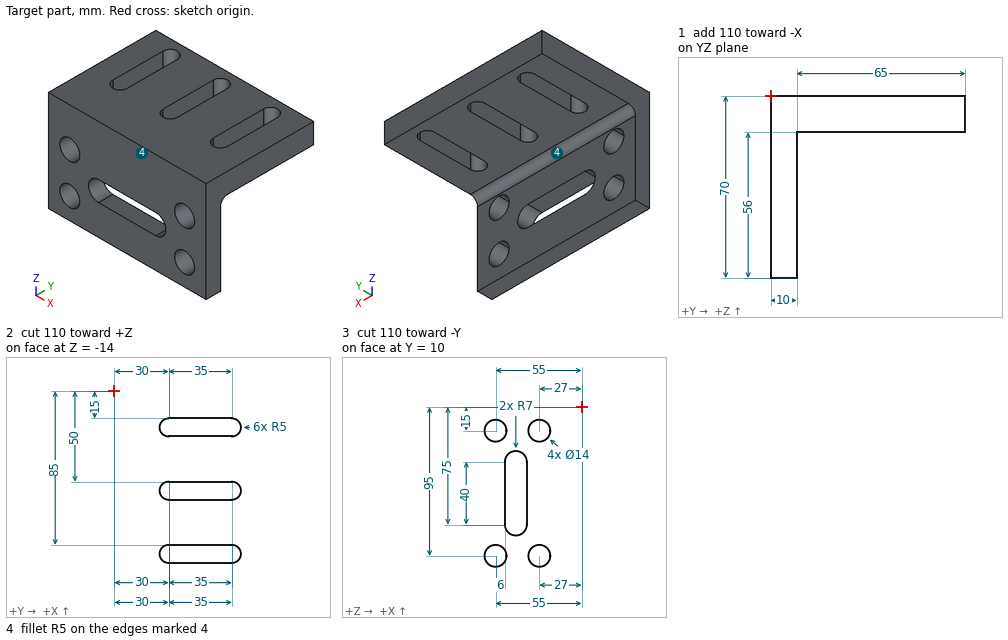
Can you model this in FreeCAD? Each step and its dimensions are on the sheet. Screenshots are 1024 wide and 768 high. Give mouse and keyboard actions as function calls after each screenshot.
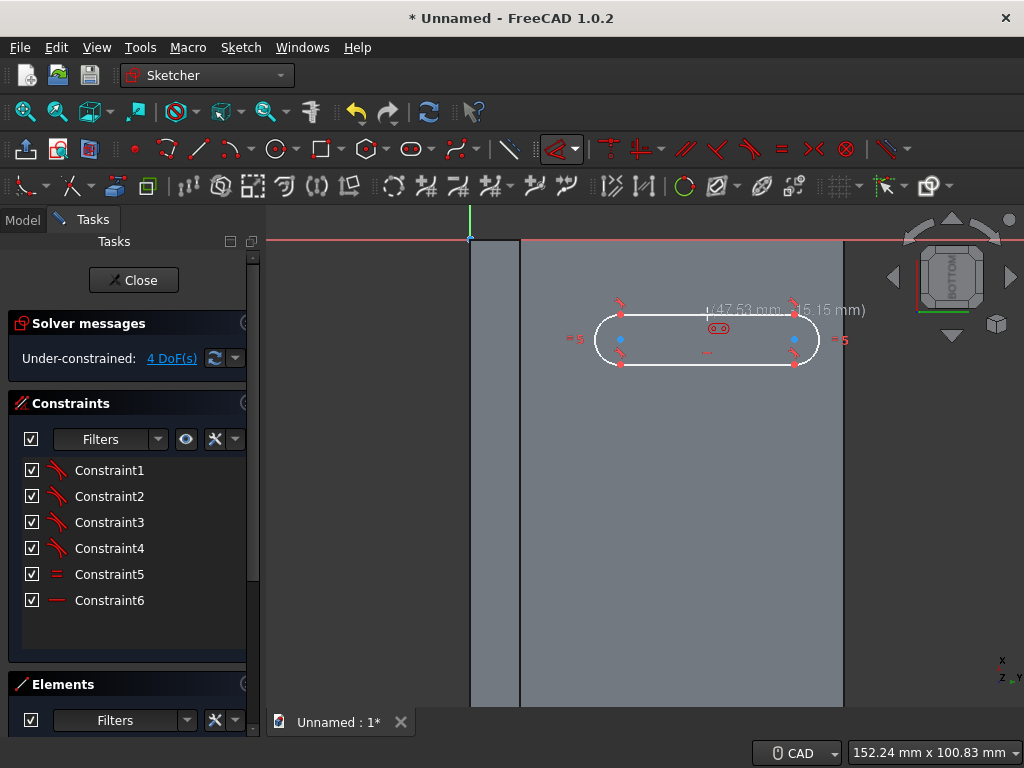
click(620, 513)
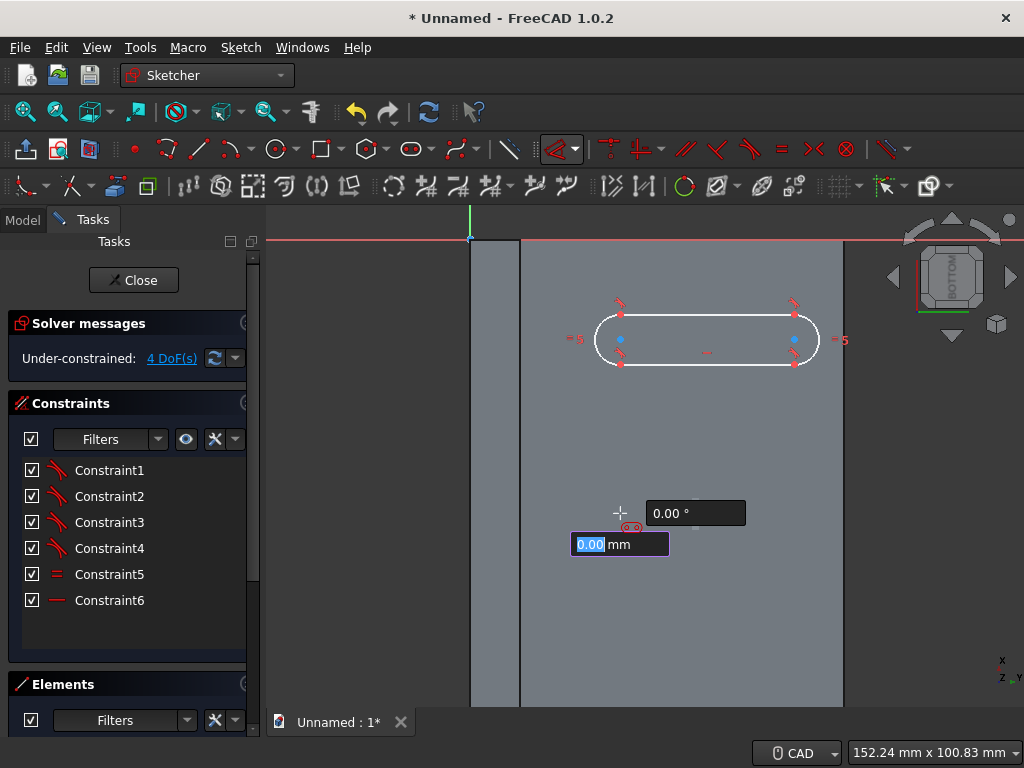
click(794, 513)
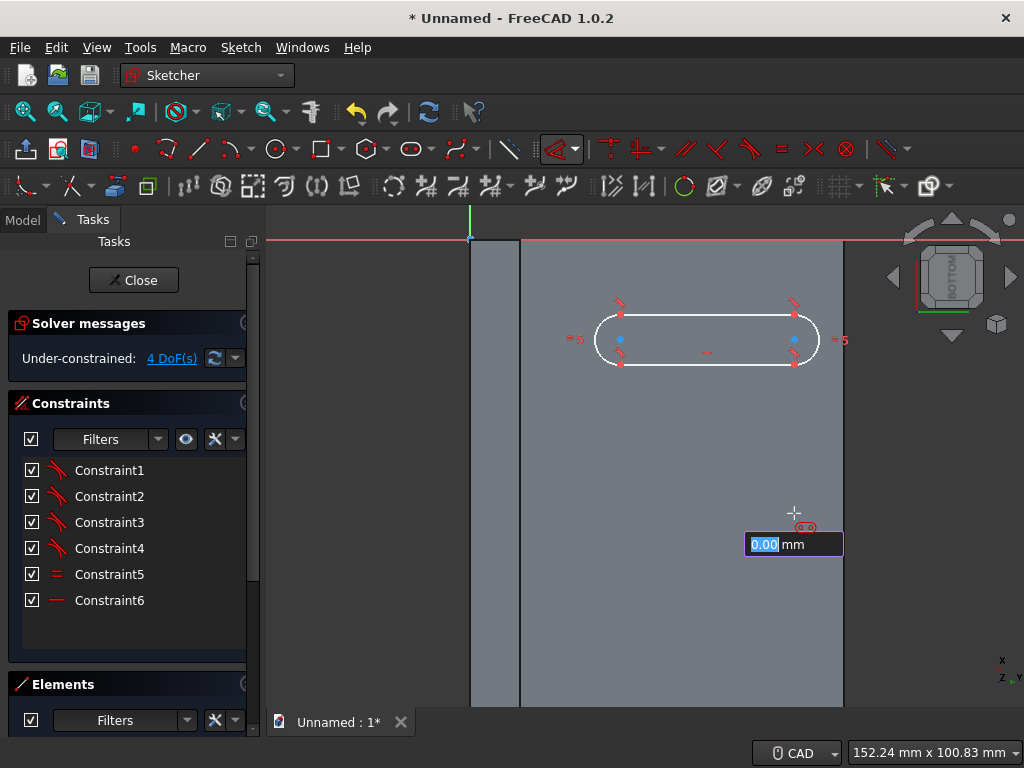
click(707, 489)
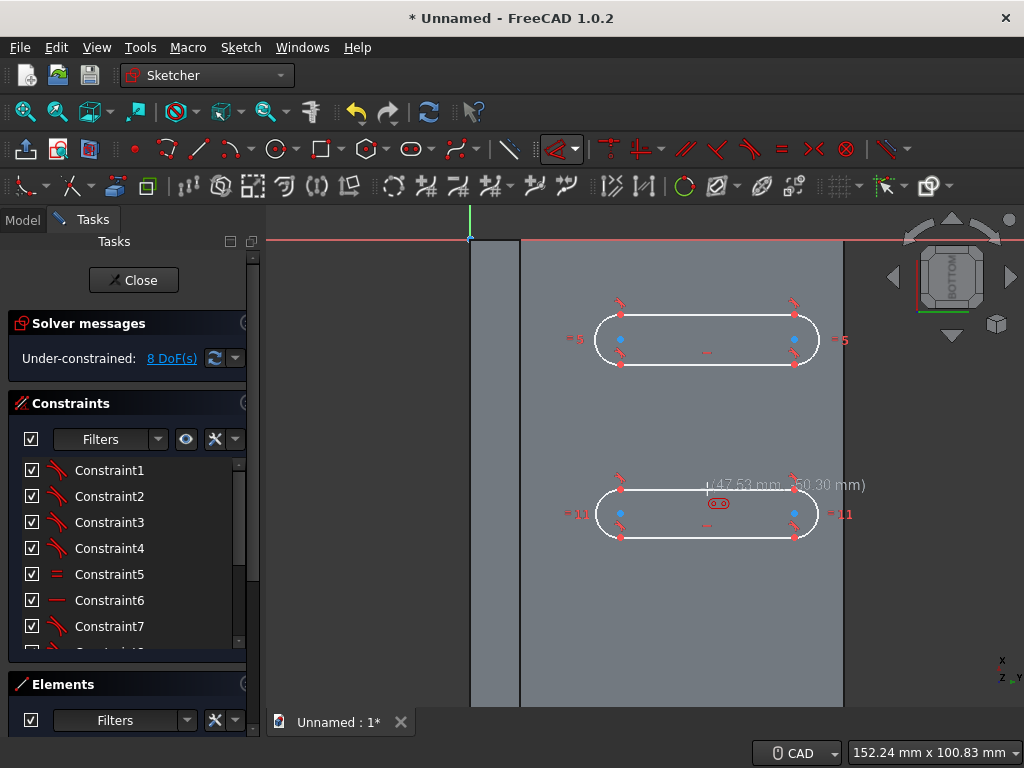
scroll(438, 415, down, 2)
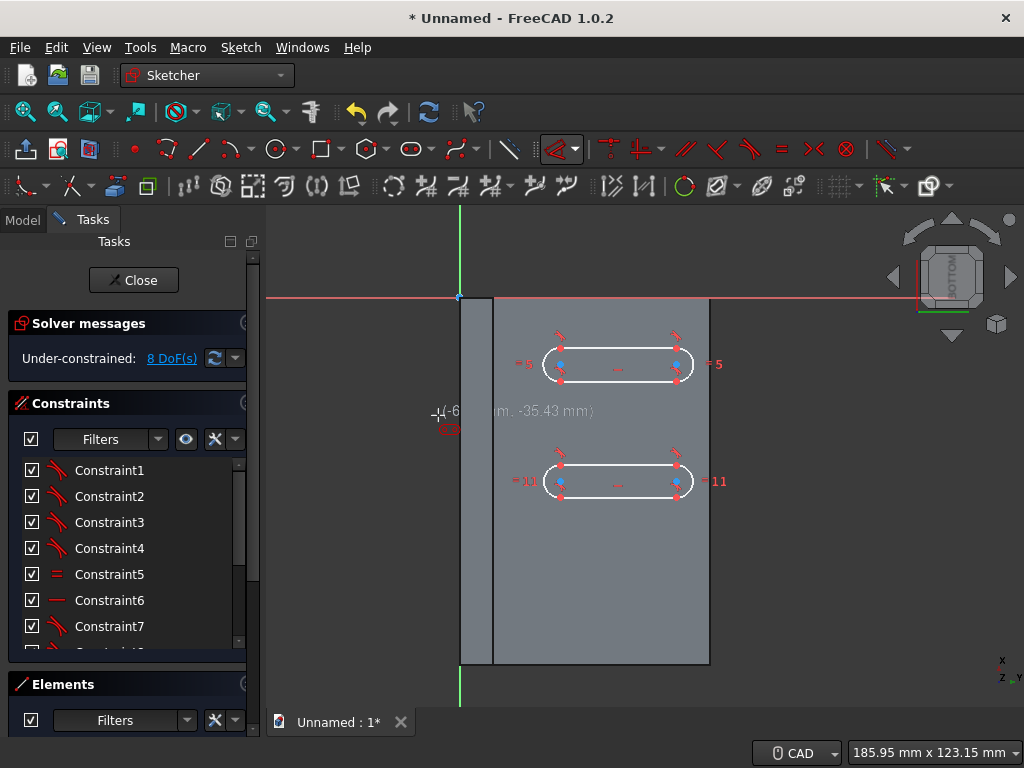
scroll(560, 598, up, 2)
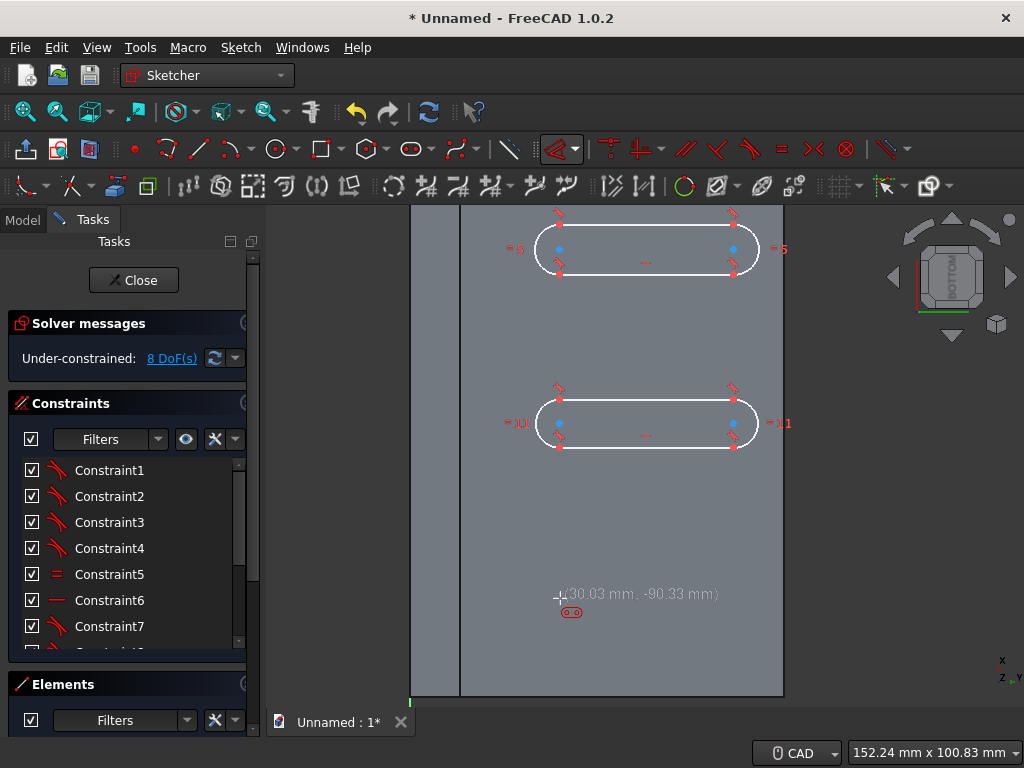
click(560, 597)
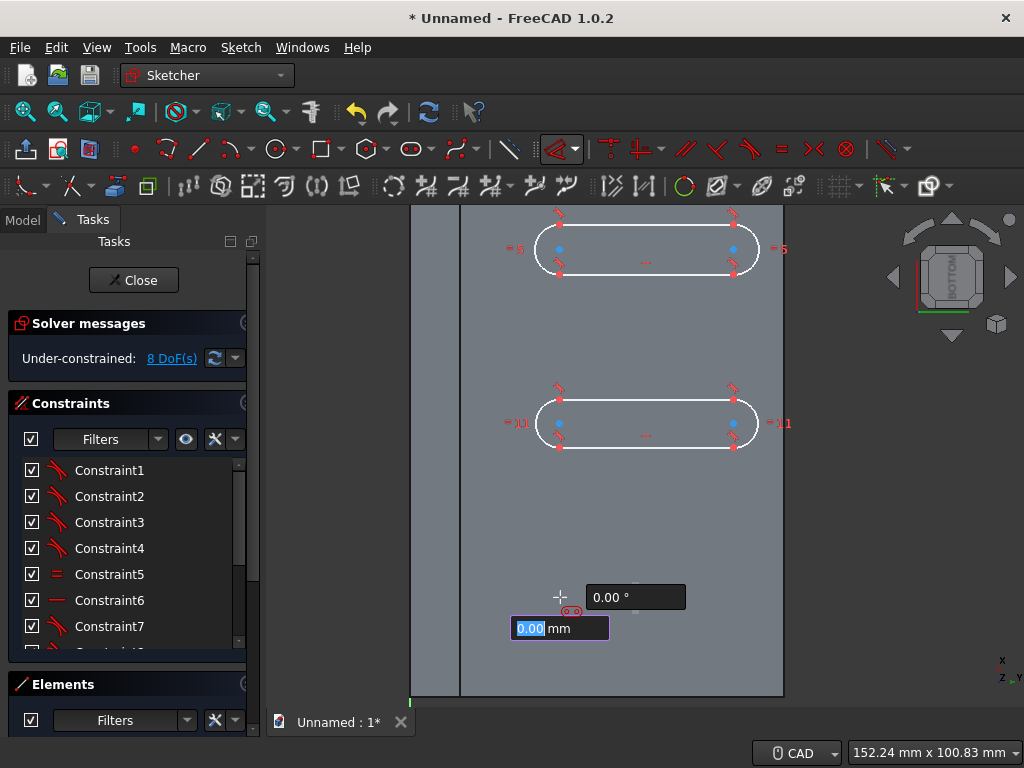
click(734, 597)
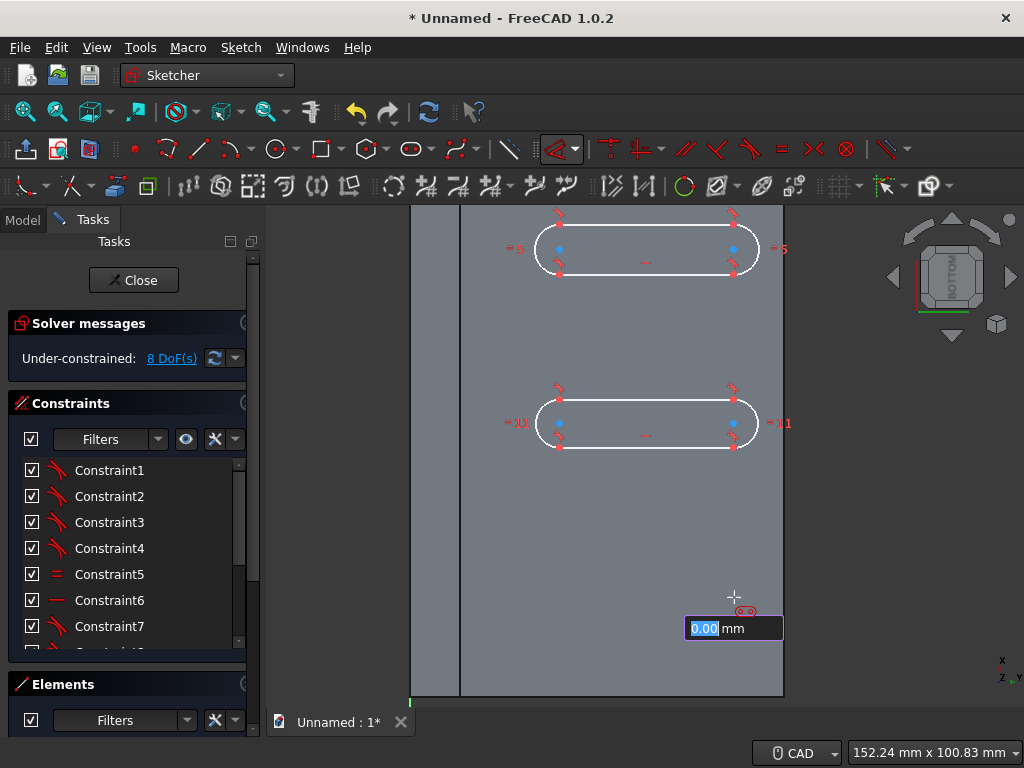
click(647, 573)
key(Escape)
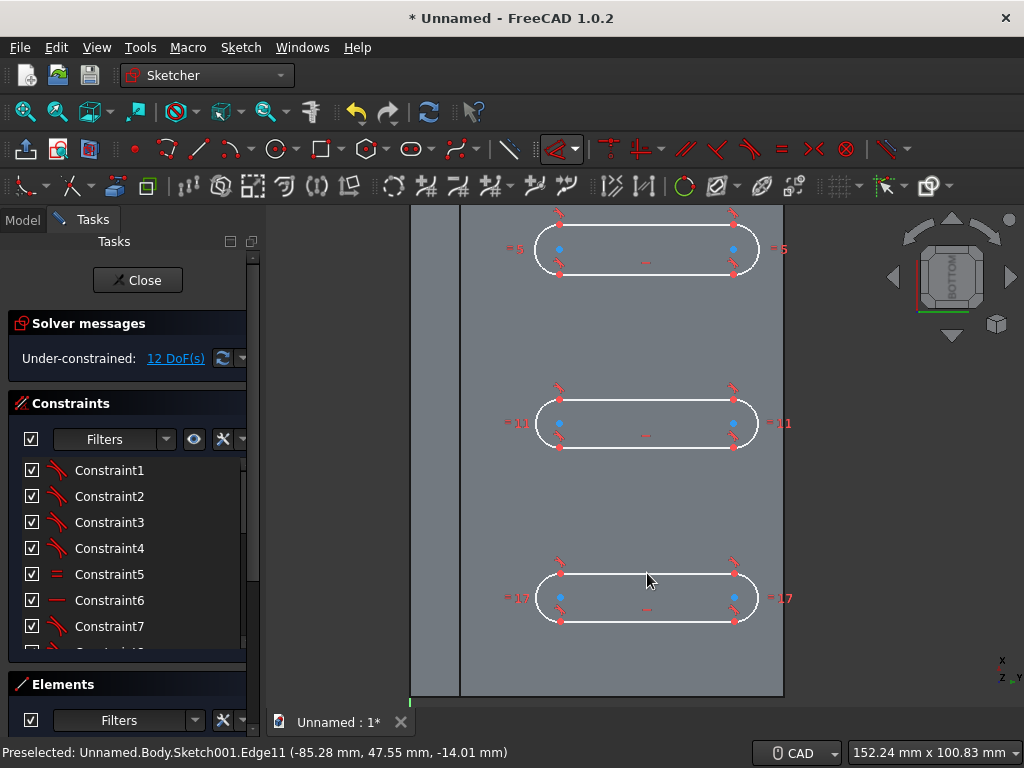
click(540, 235)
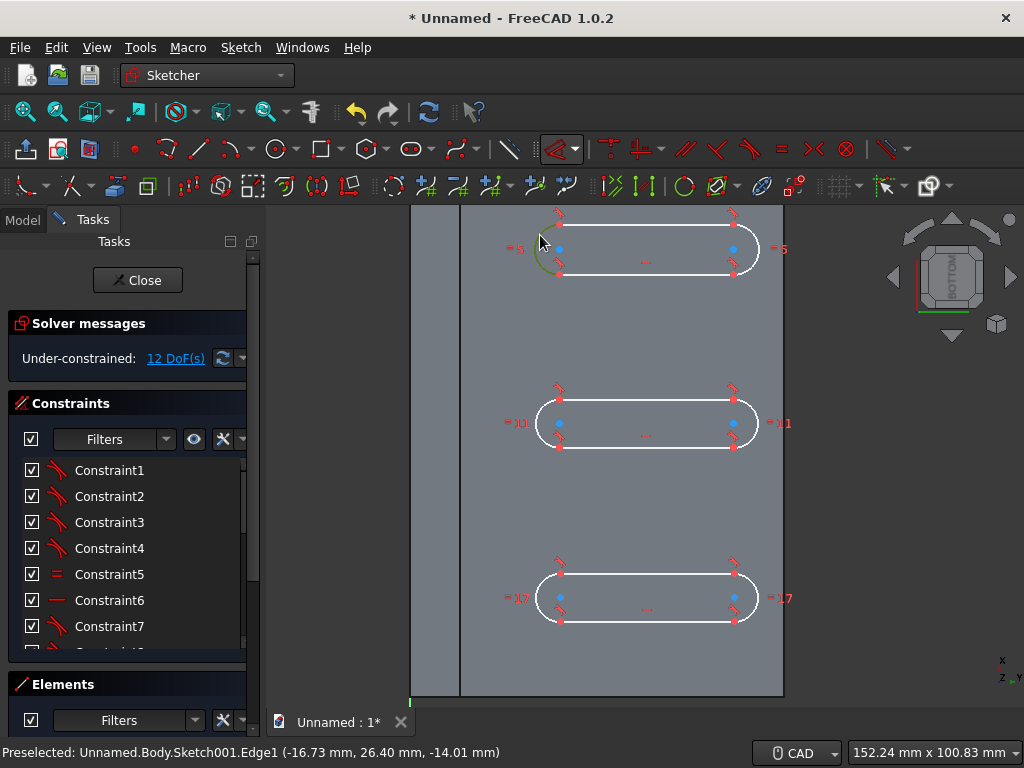
click(541, 410)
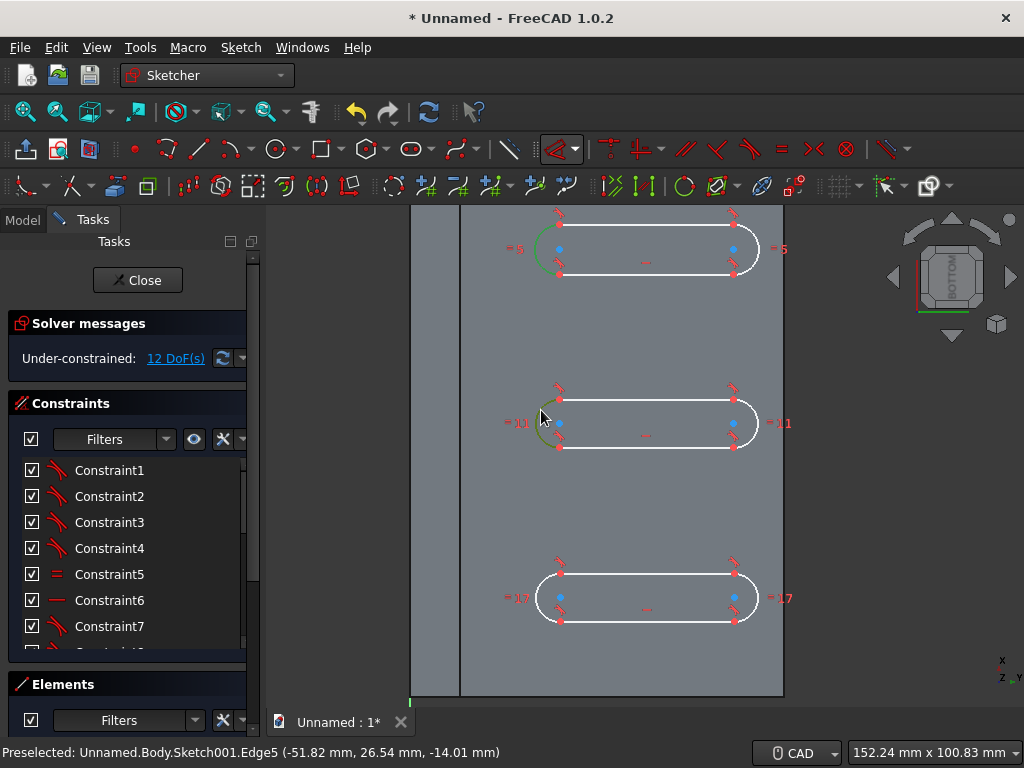
click(541, 584)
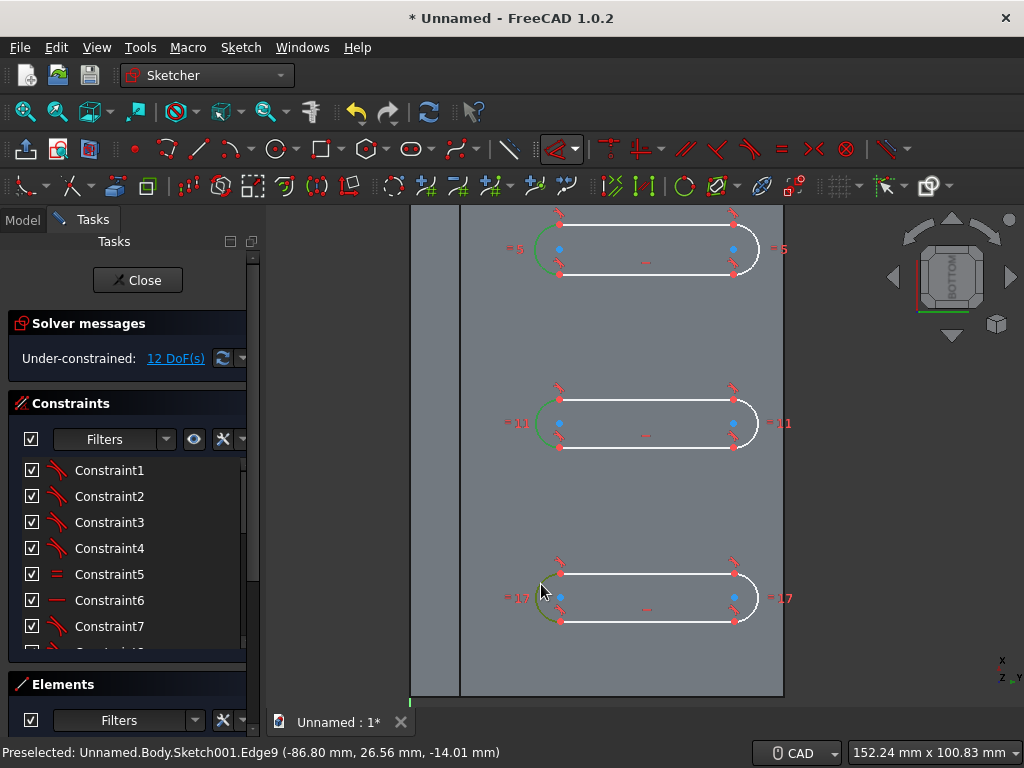
click(782, 150)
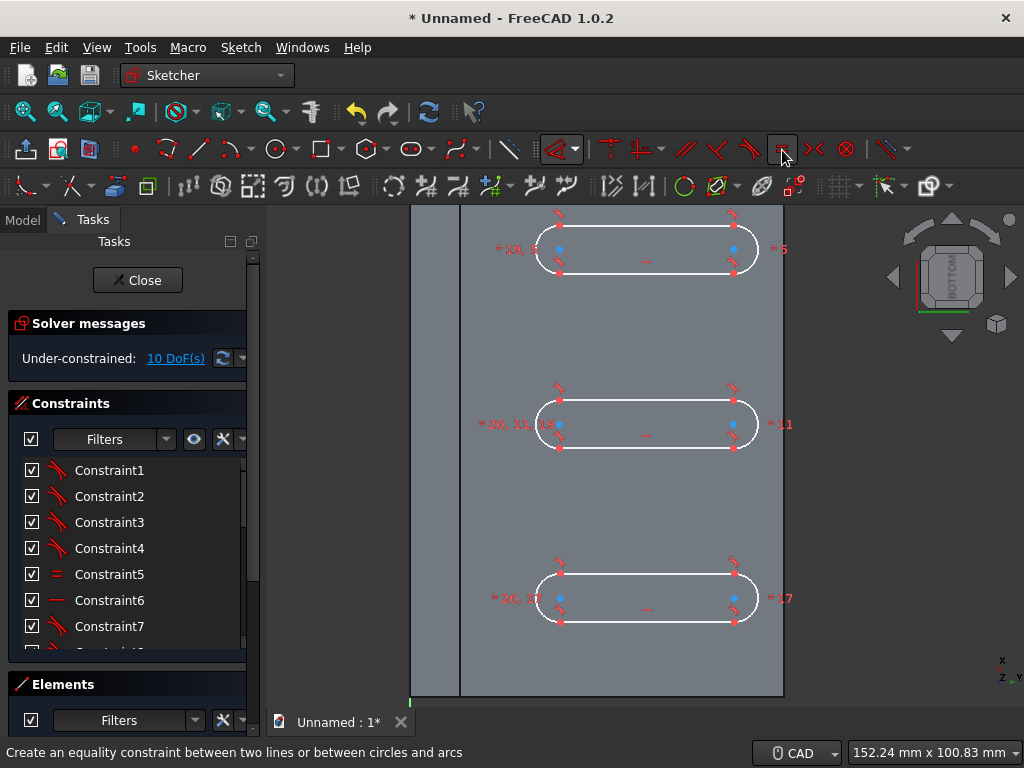
scroll(540, 236, up, 3)